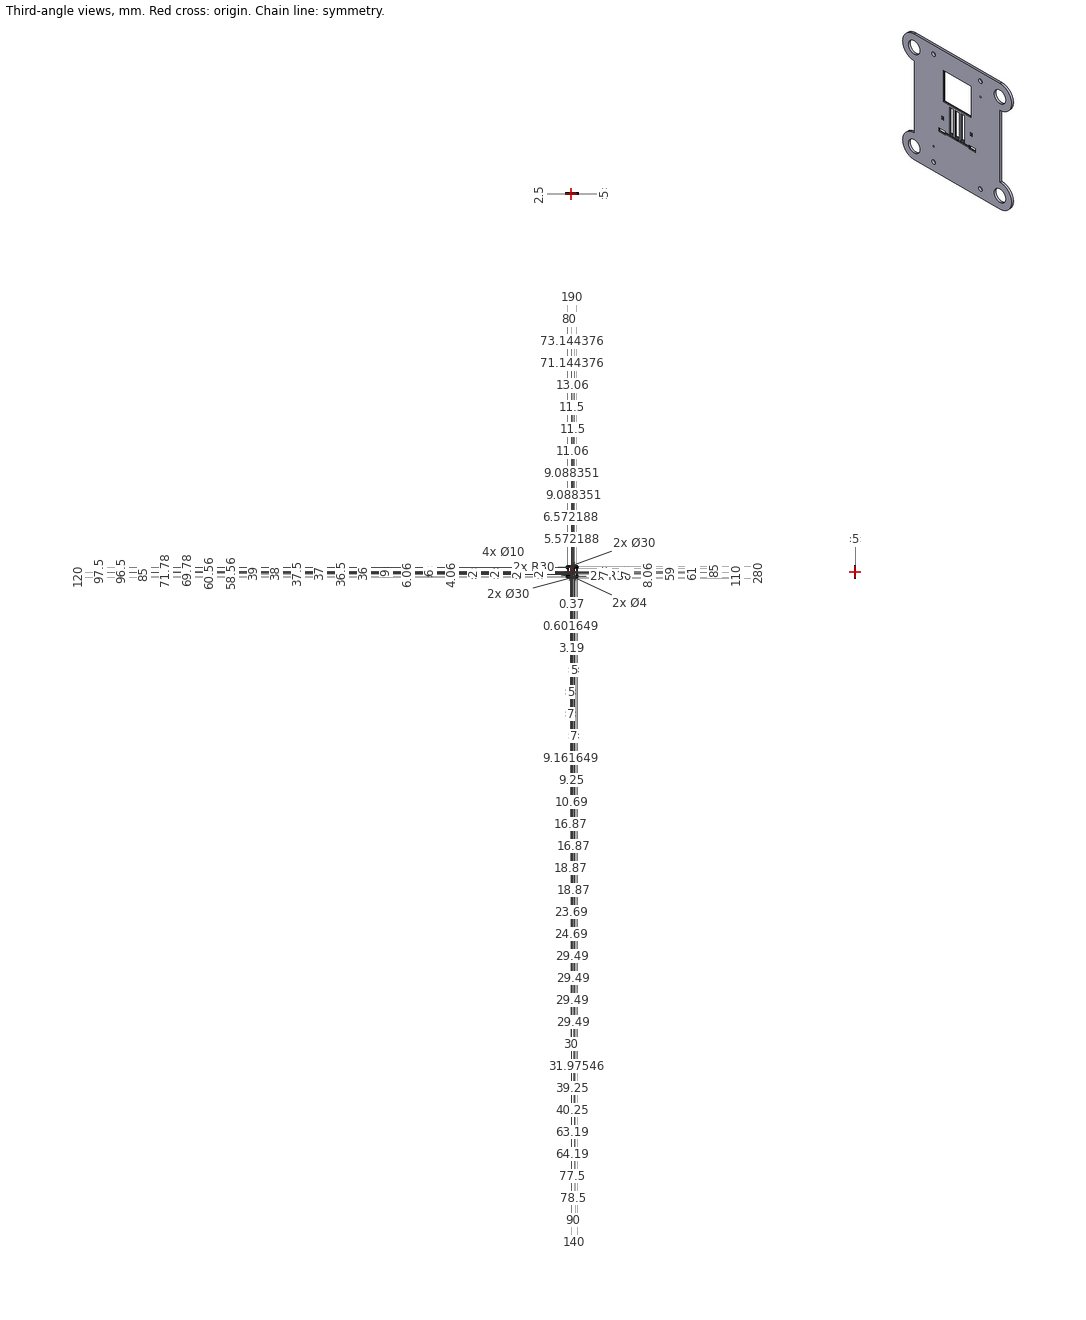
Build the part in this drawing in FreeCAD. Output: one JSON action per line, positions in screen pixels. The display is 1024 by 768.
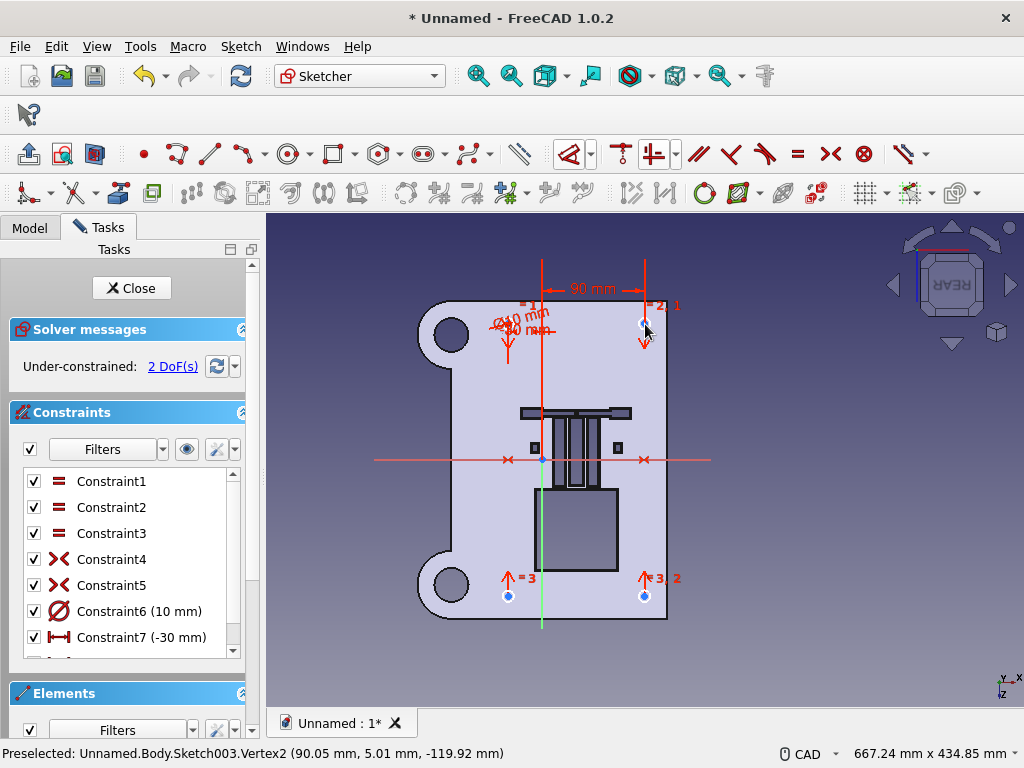
{"action": "left_click", "coordinate": [508, 324]}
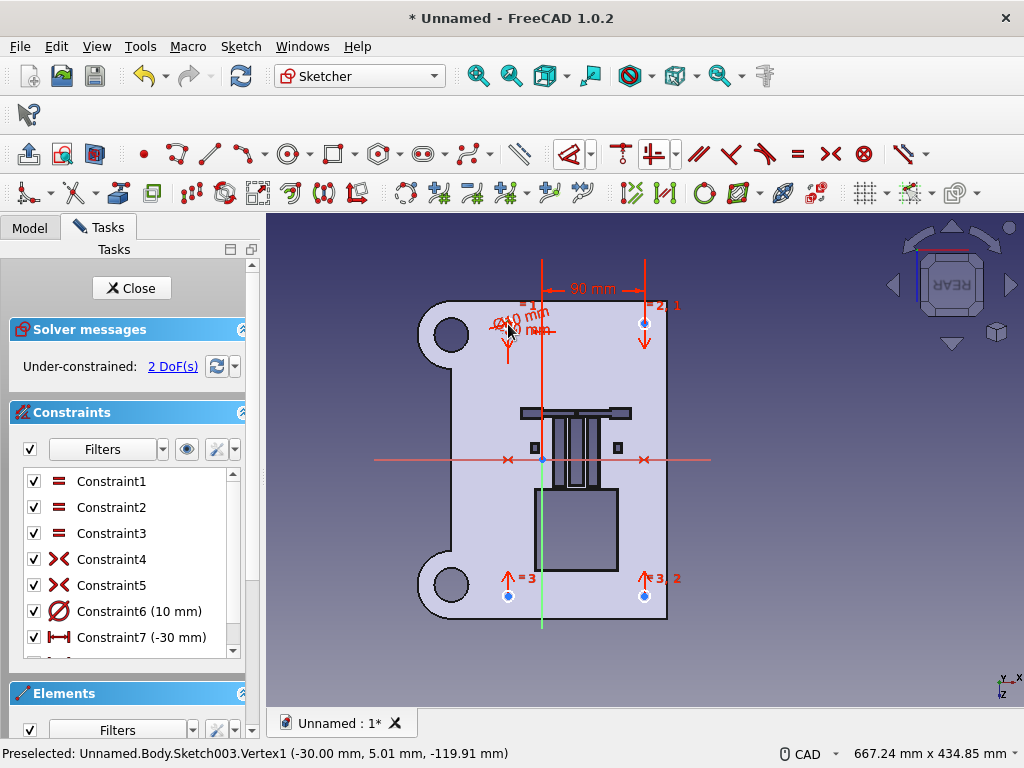
{"action": "left_click", "coordinate": [590, 154]}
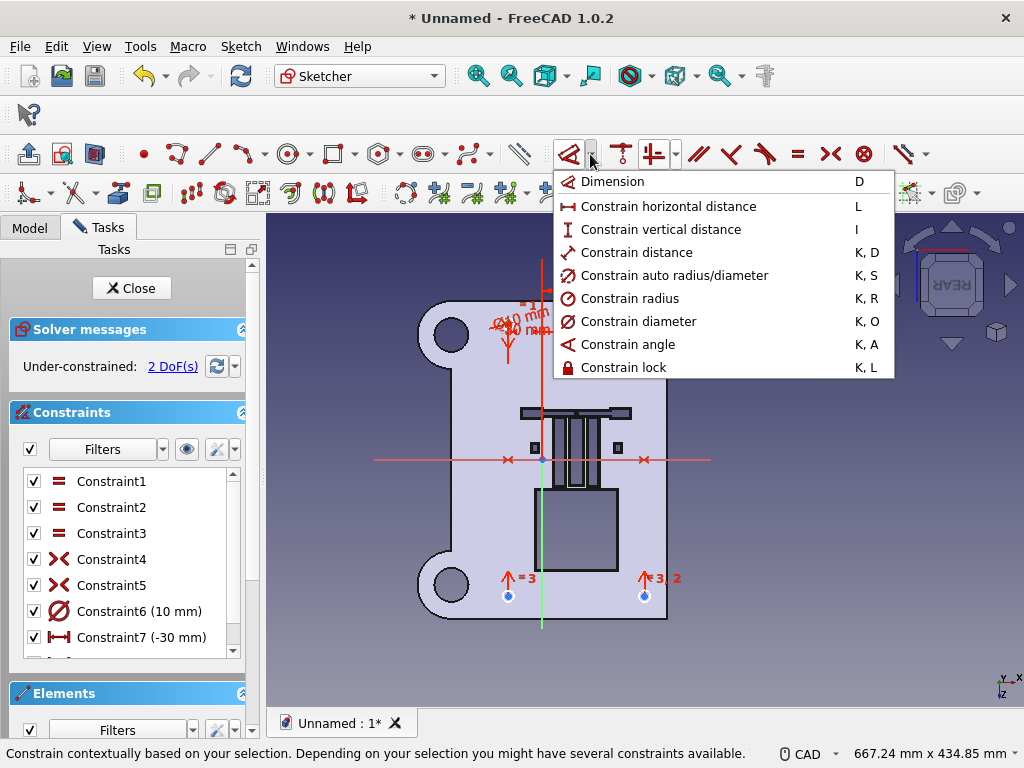
{"action": "left_click", "coordinate": [724, 230]}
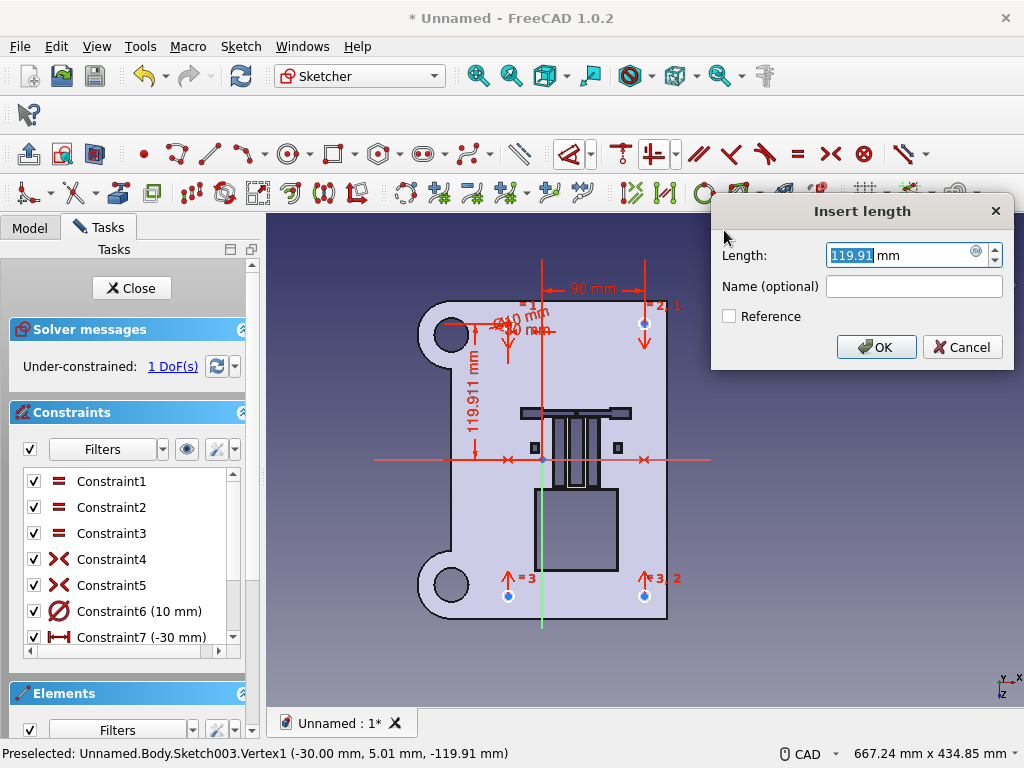
{"action": "type", "text": "120"}
{"action": "key", "text": "Return"}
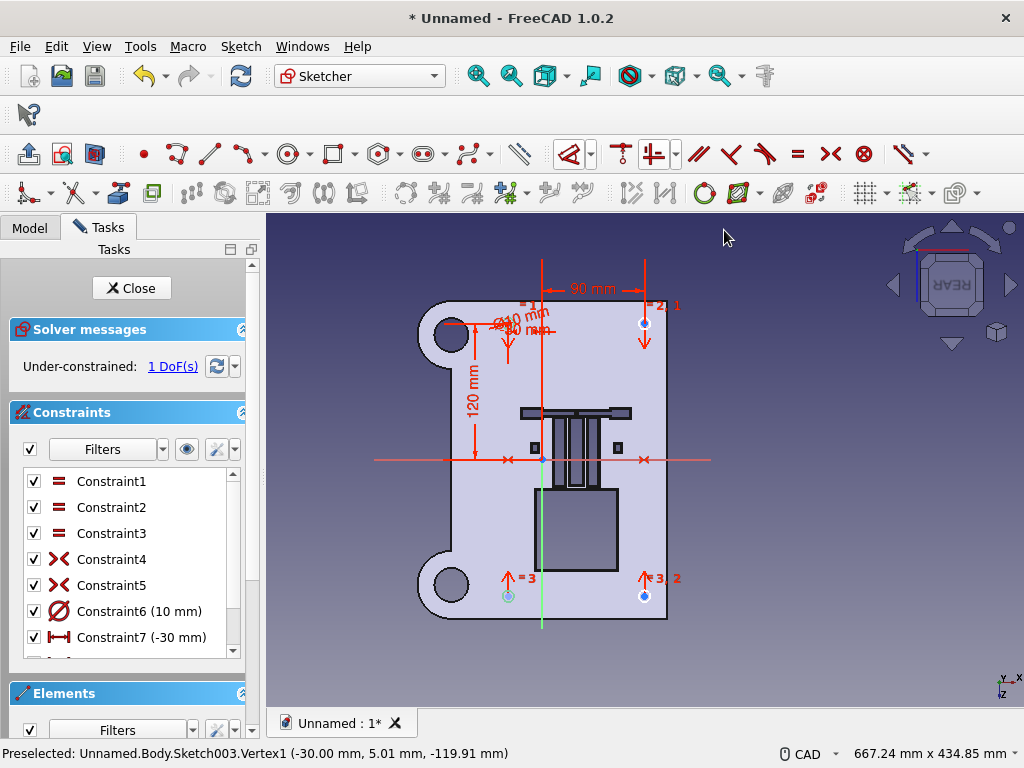
{"action": "left_click", "coordinate": [645, 324]}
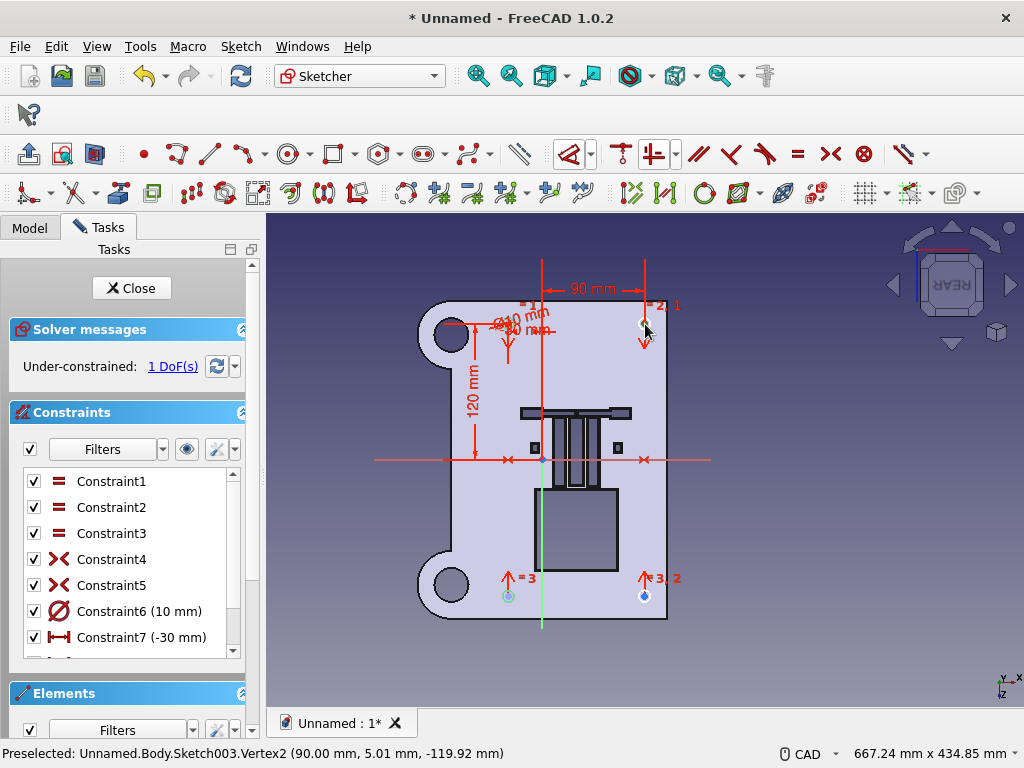
{"action": "left_click", "coordinate": [590, 154]}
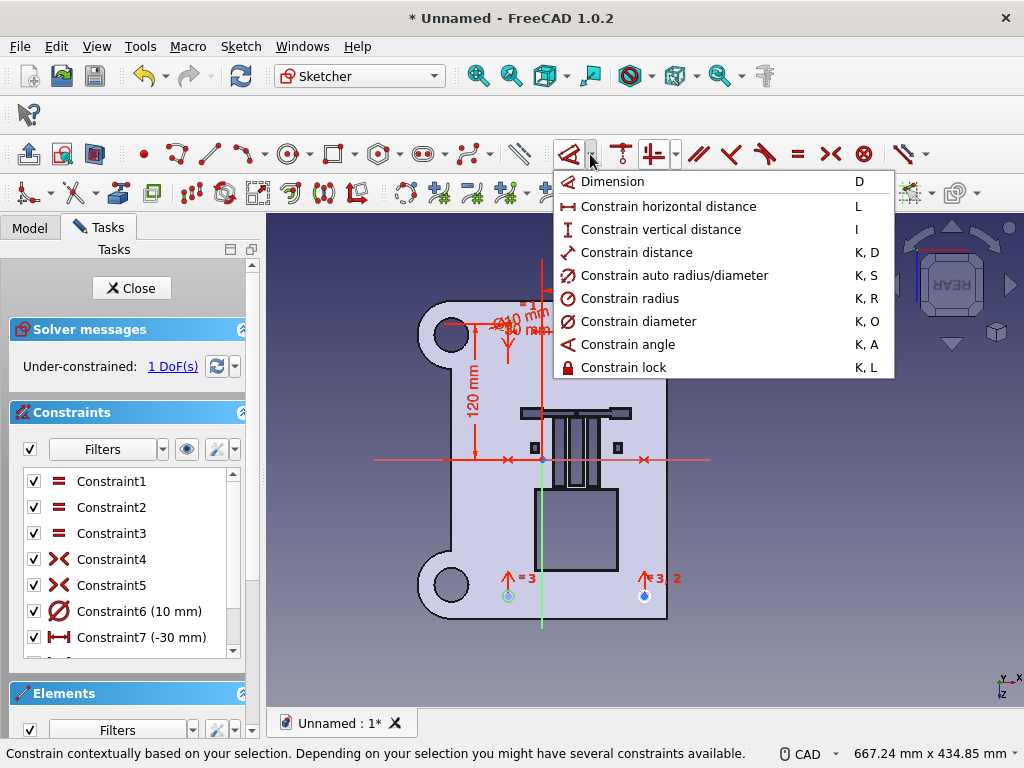
{"action": "left_click", "coordinate": [724, 230]}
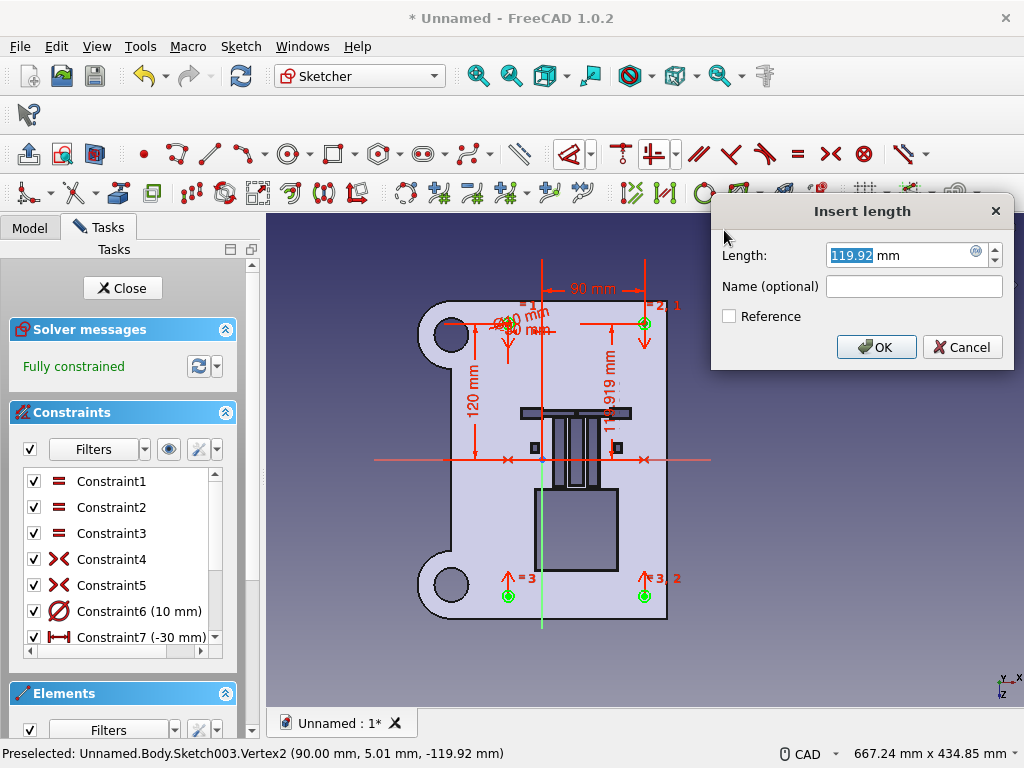
{"action": "type", "text": "120"}
{"action": "key", "text": "Return"}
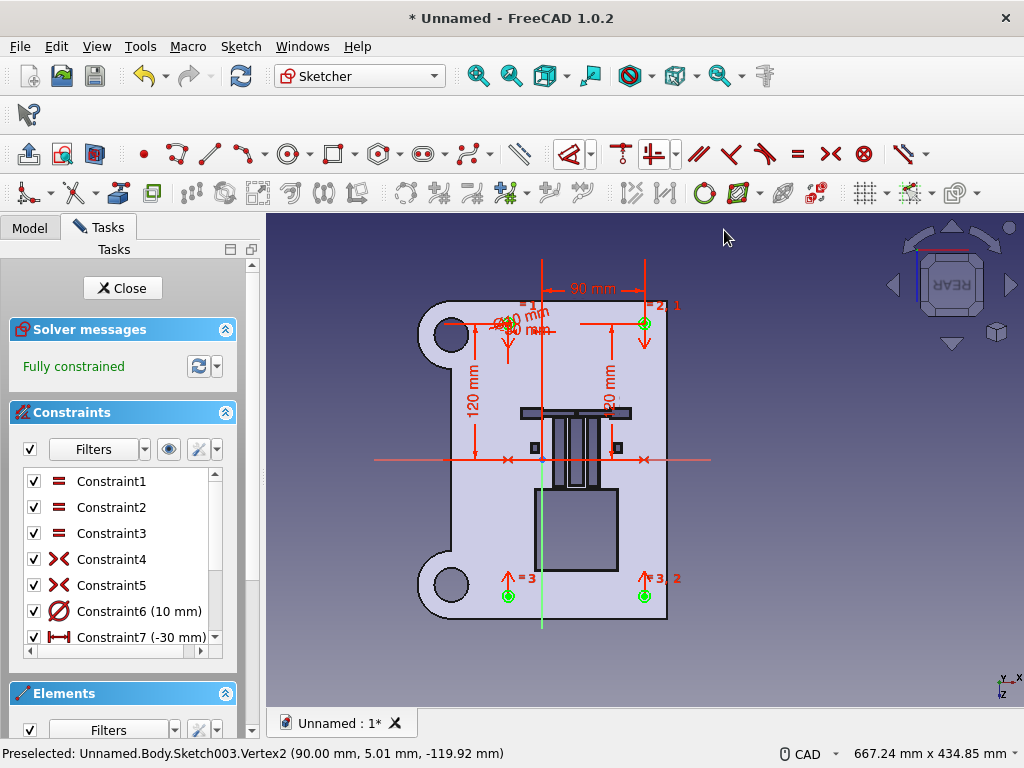
{"action": "left_click", "coordinate": [123, 288]}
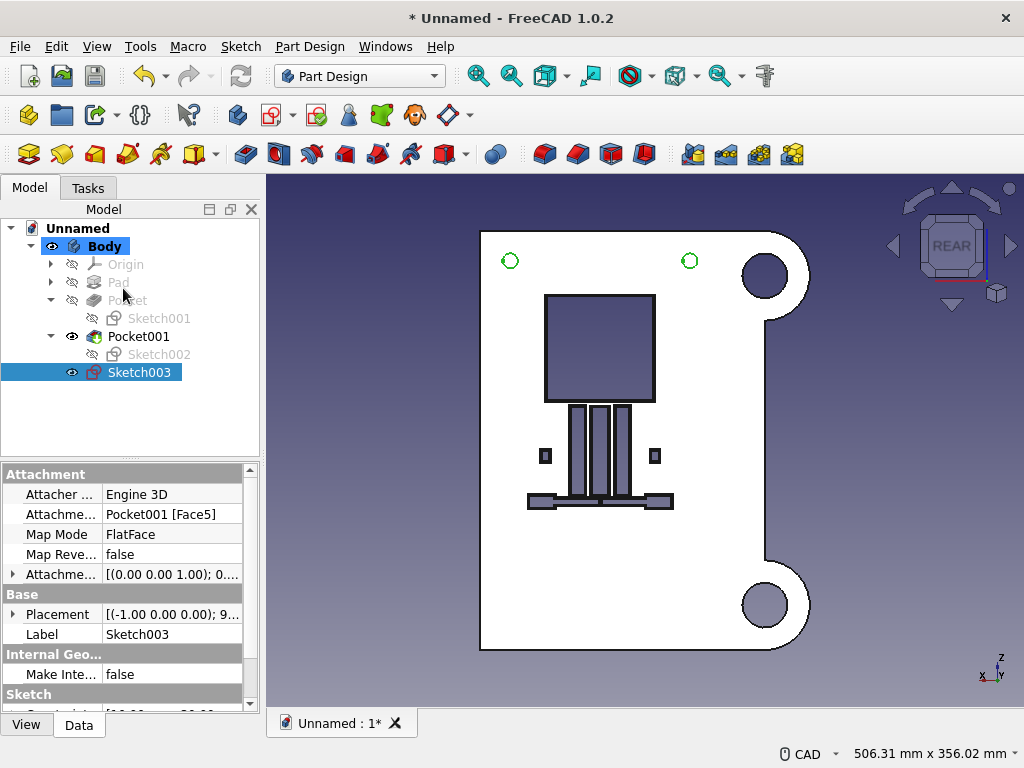
{"action": "left_click", "coordinate": [246, 154]}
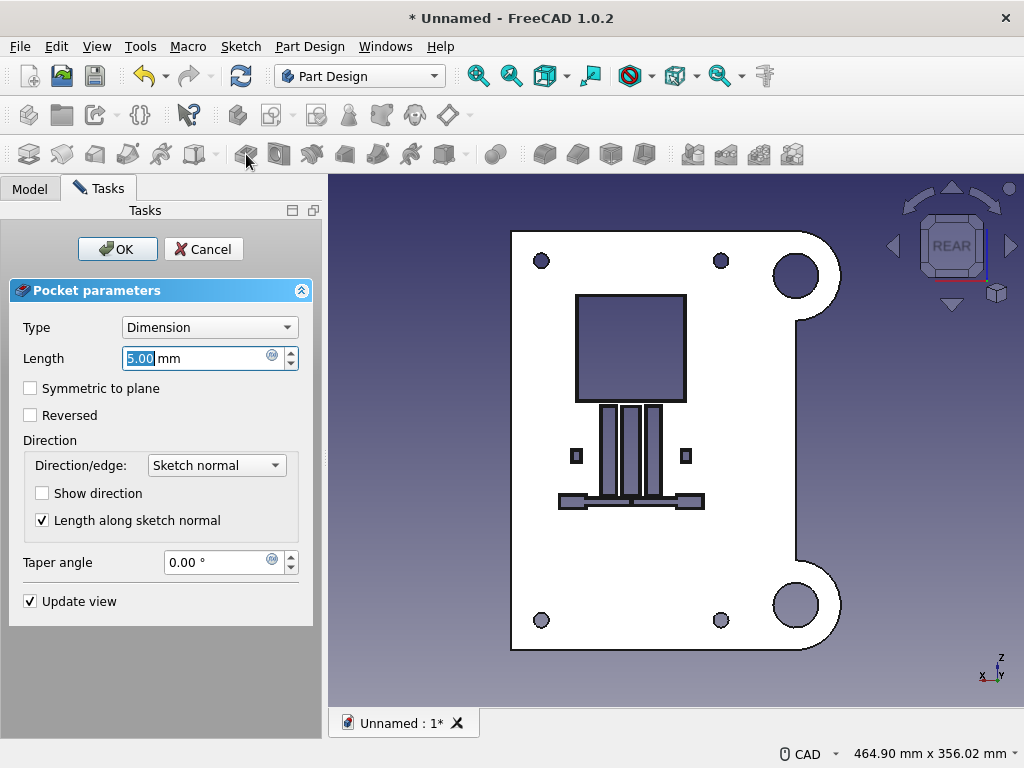
{"action": "left_click", "coordinate": [210, 328]}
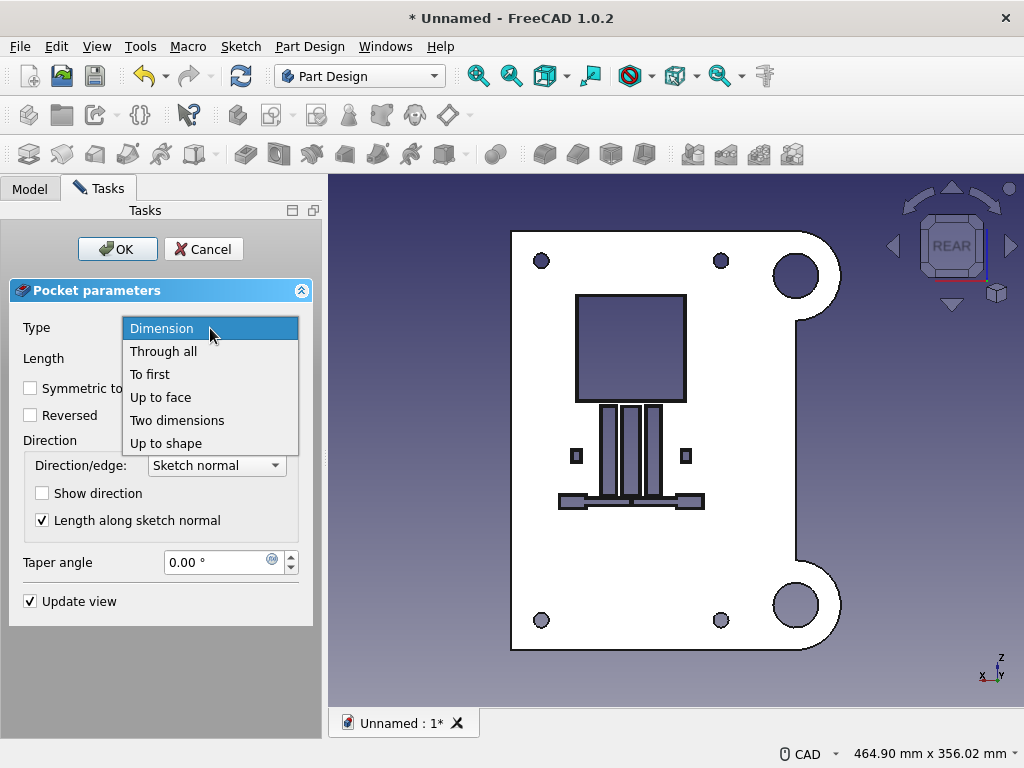
{"action": "left_click", "coordinate": [208, 352]}